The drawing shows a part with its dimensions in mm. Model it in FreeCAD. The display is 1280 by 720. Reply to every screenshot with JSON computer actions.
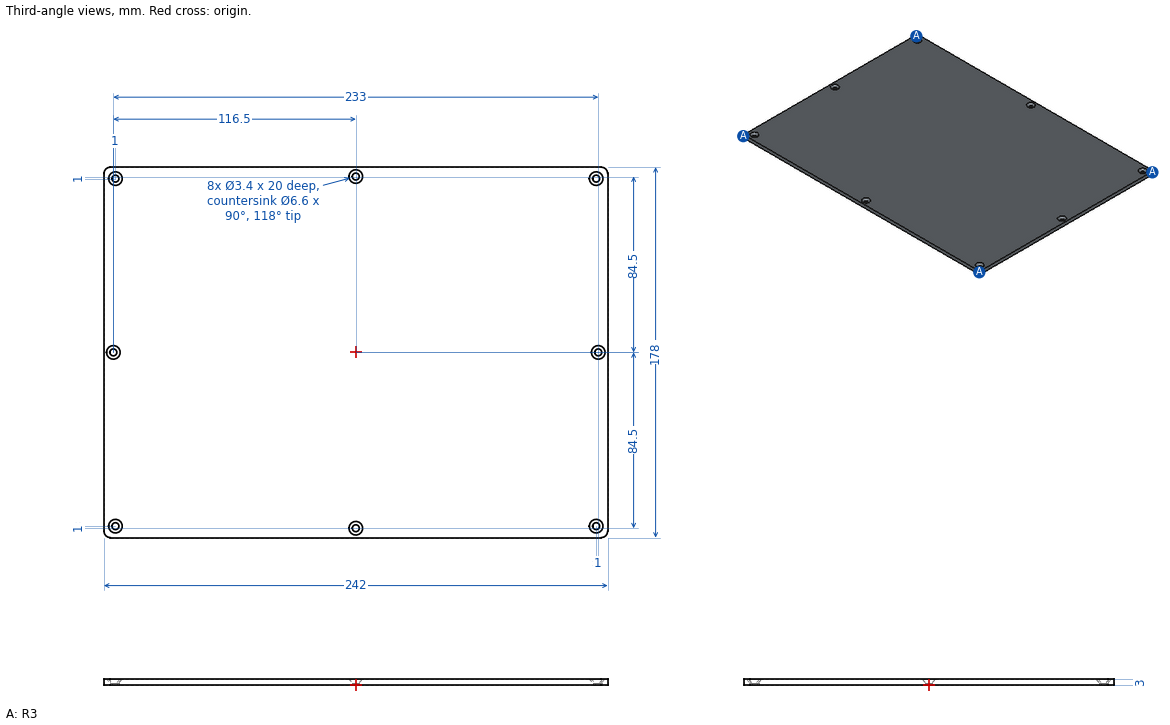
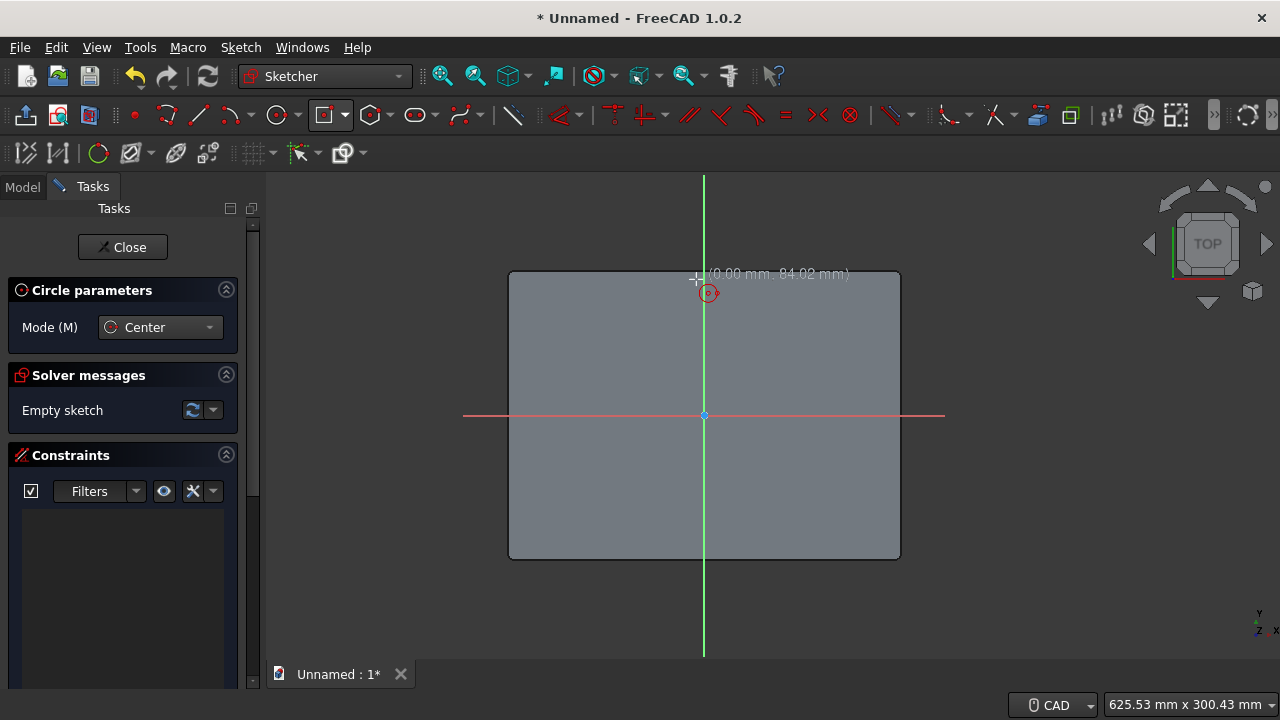
{"action": "left_click", "coordinate": [704, 279]}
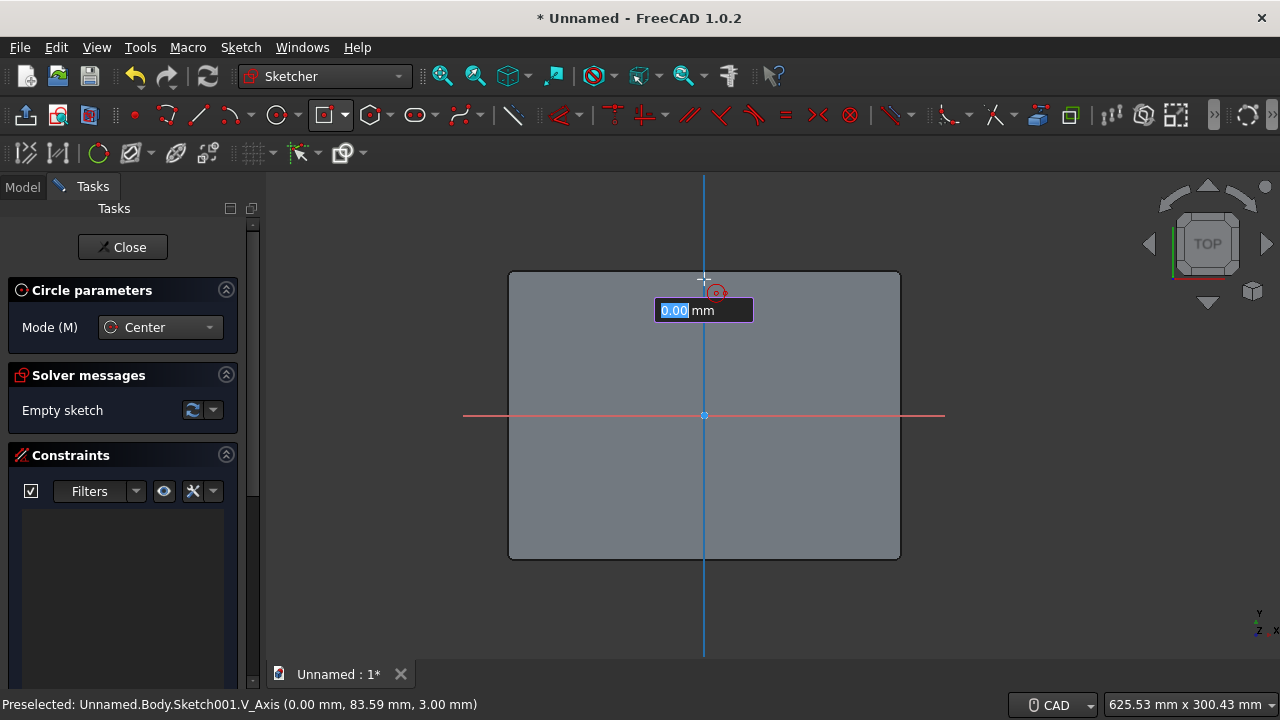
{"action": "scroll", "coordinate": [707, 278], "scroll_direction": "up", "scroll_amount": 10}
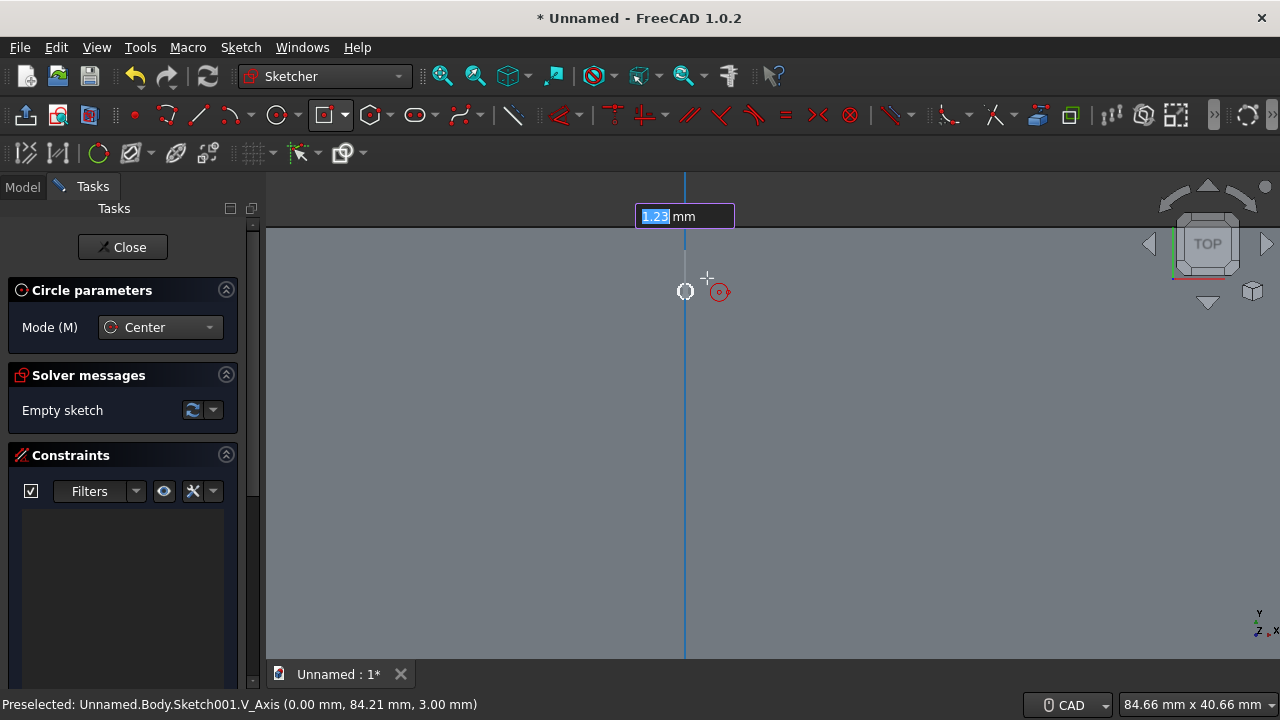
{"action": "left_click", "coordinate": [705, 274]}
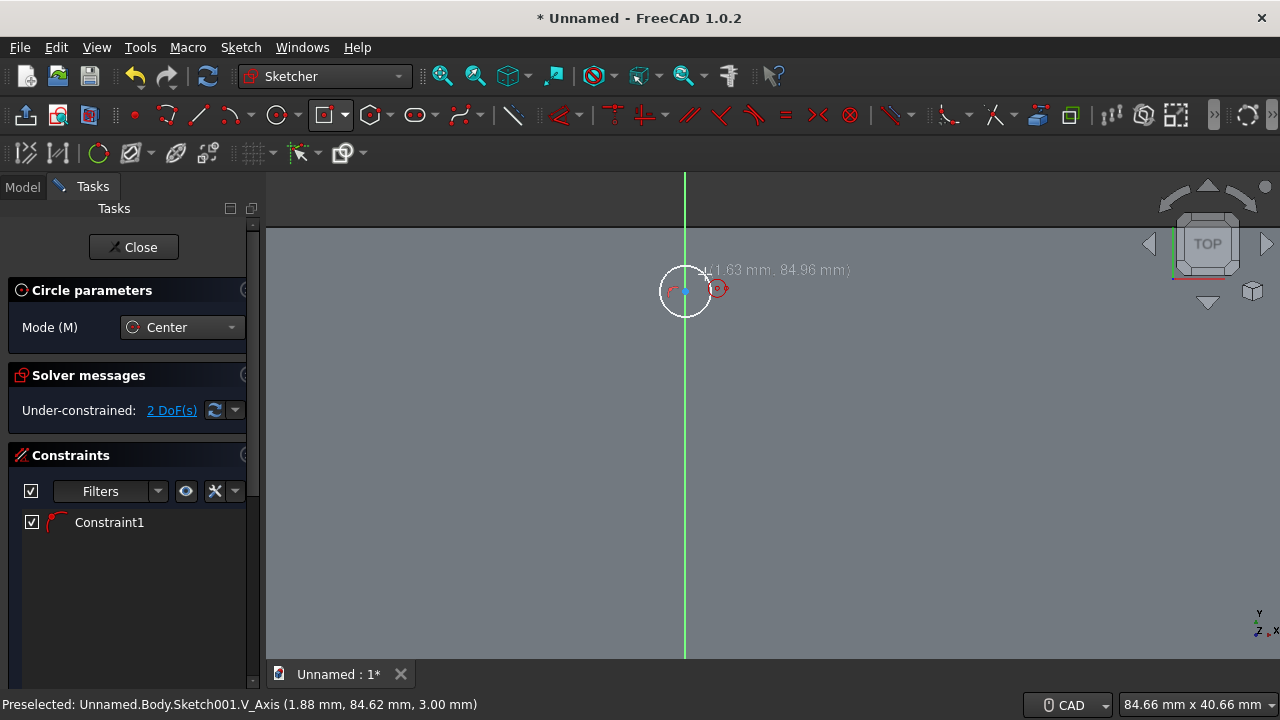
{"action": "scroll", "coordinate": [707, 278], "scroll_direction": "down", "scroll_amount": 10}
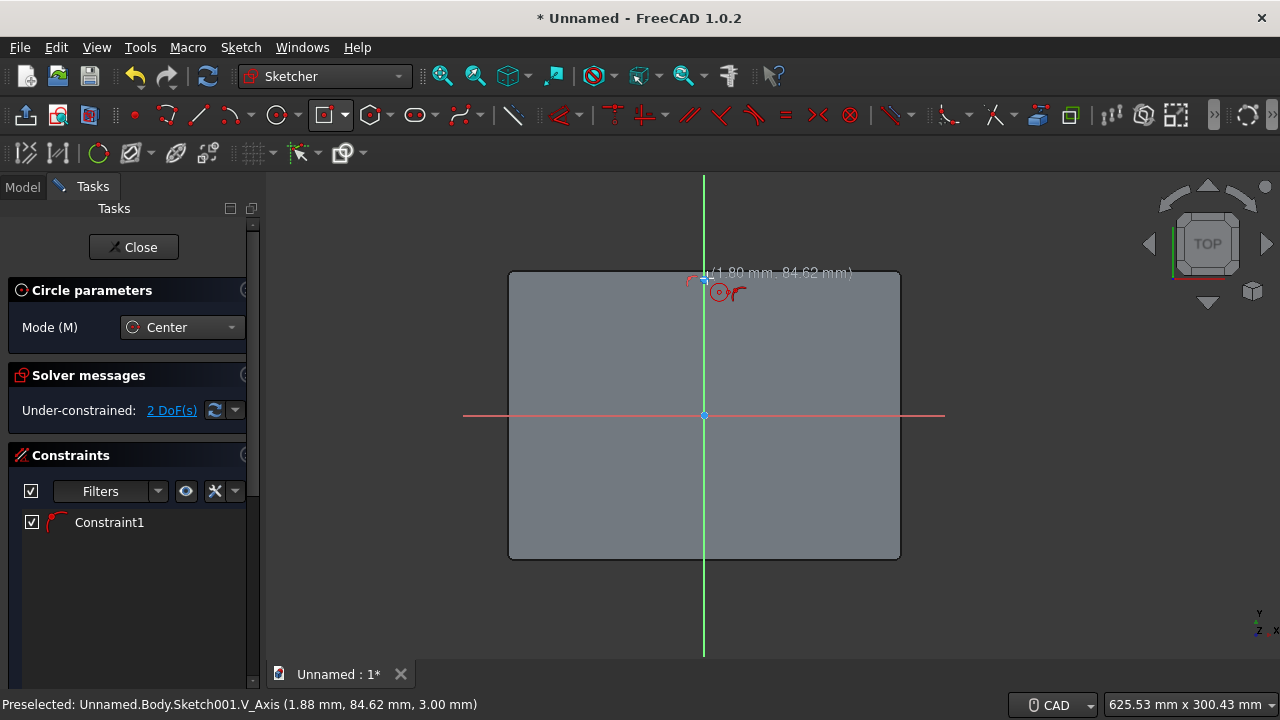
{"action": "scroll", "coordinate": [516, 415], "scroll_direction": "up", "scroll_amount": 11}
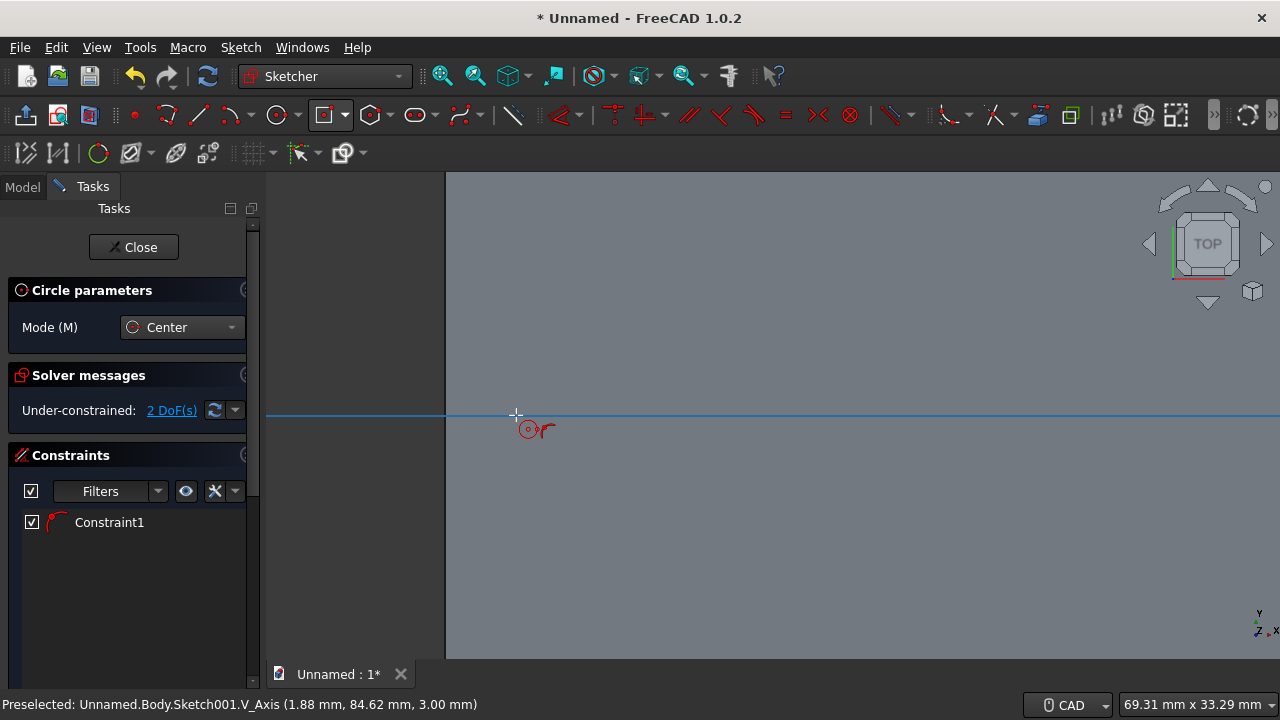
{"action": "scroll", "coordinate": [516, 416], "scroll_direction": "down", "scroll_amount": 11}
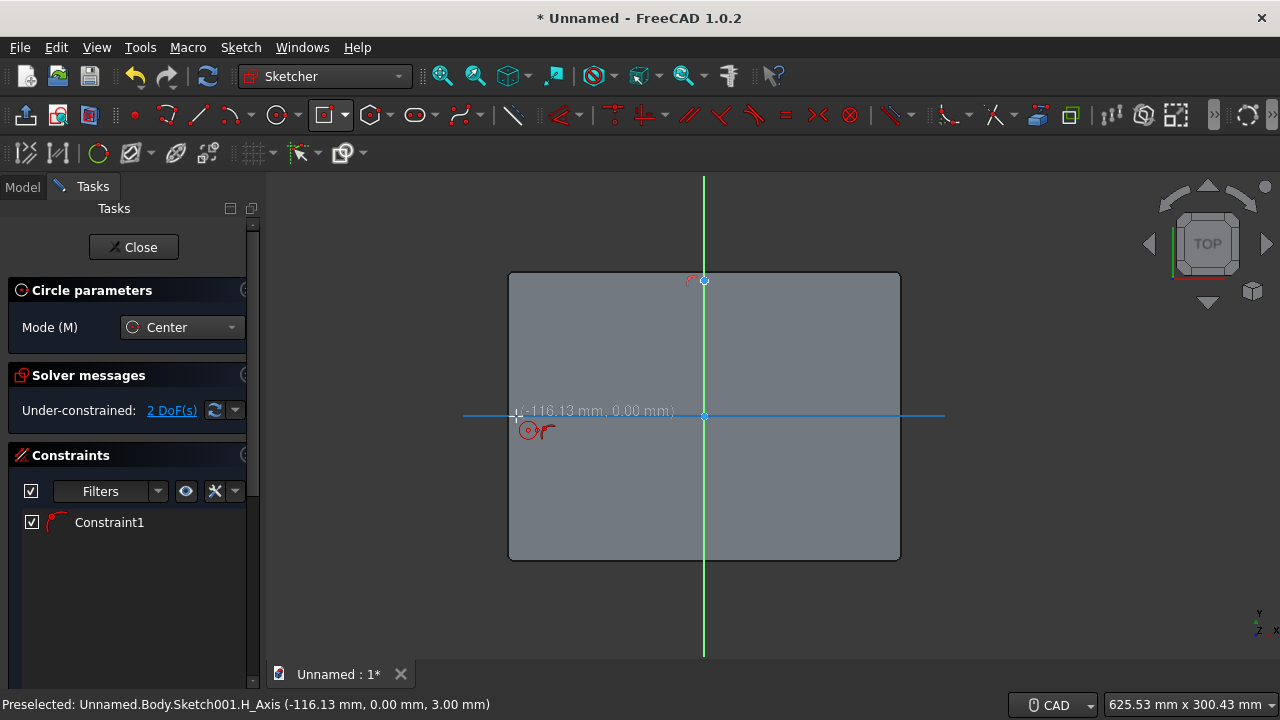
{"action": "left_click", "coordinate": [516, 416]}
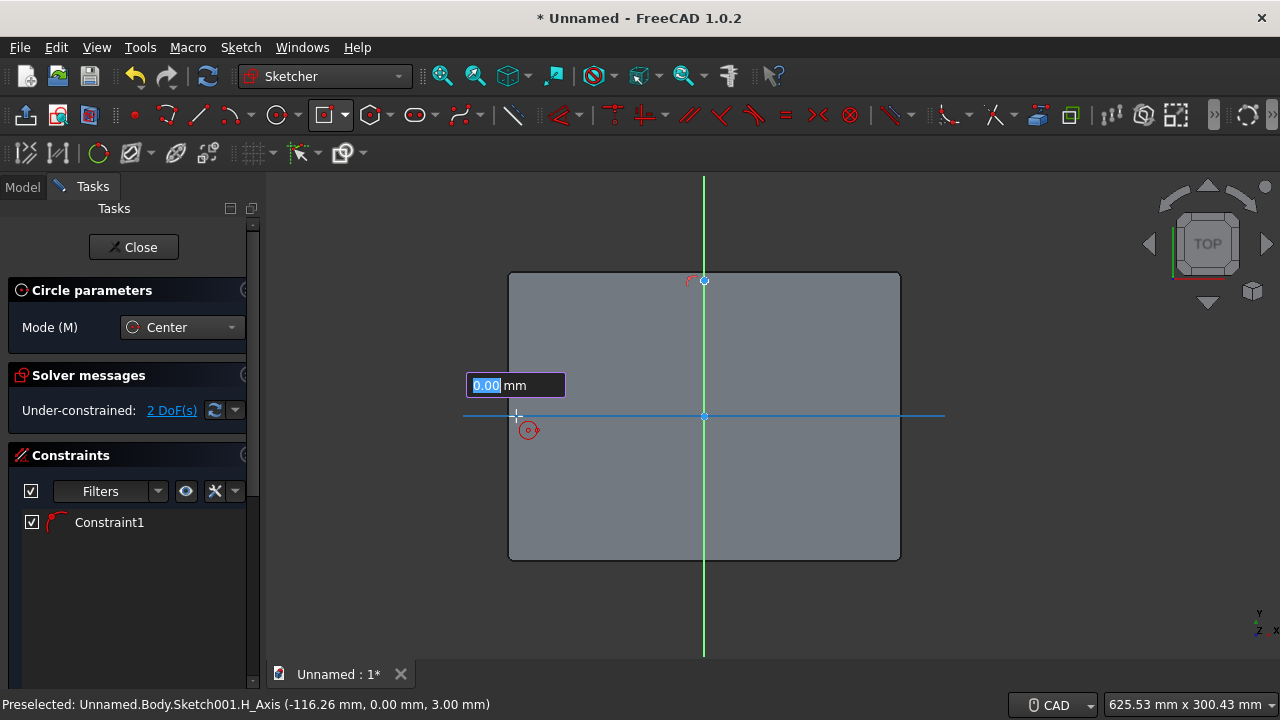
{"action": "scroll", "coordinate": [515, 419], "scroll_direction": "up", "scroll_amount": 10}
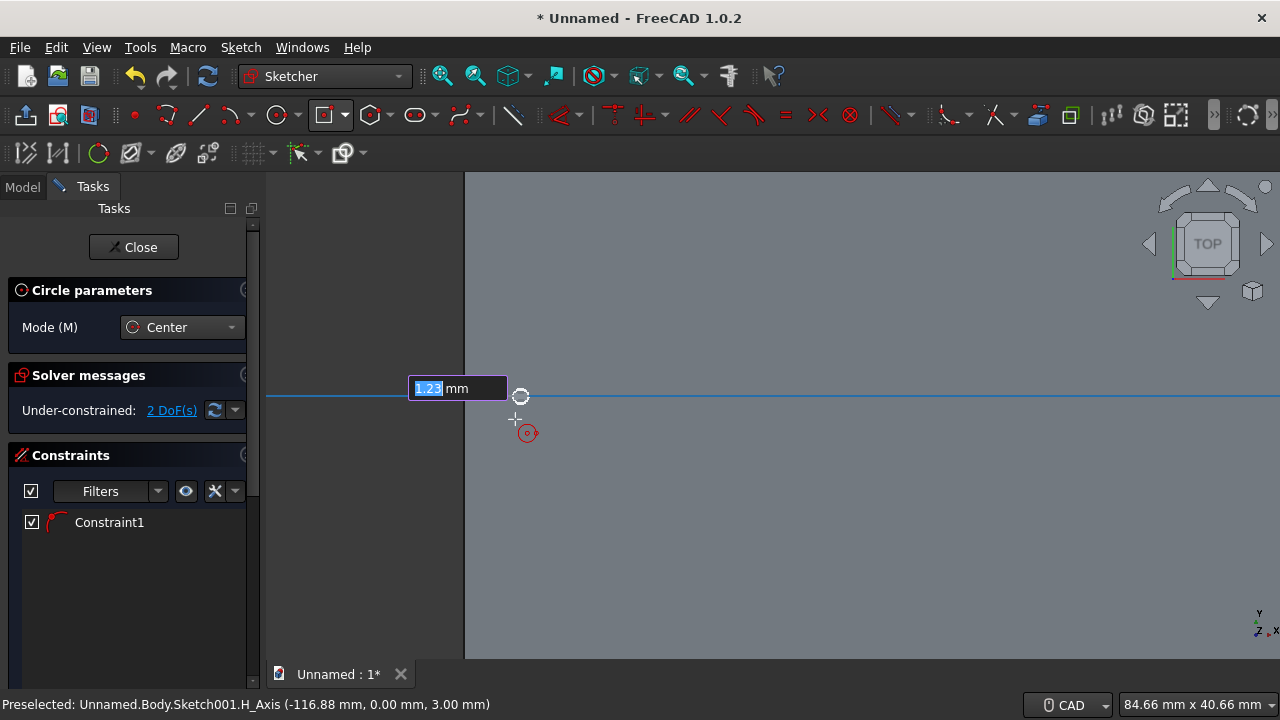
{"action": "left_click", "coordinate": [511, 416]}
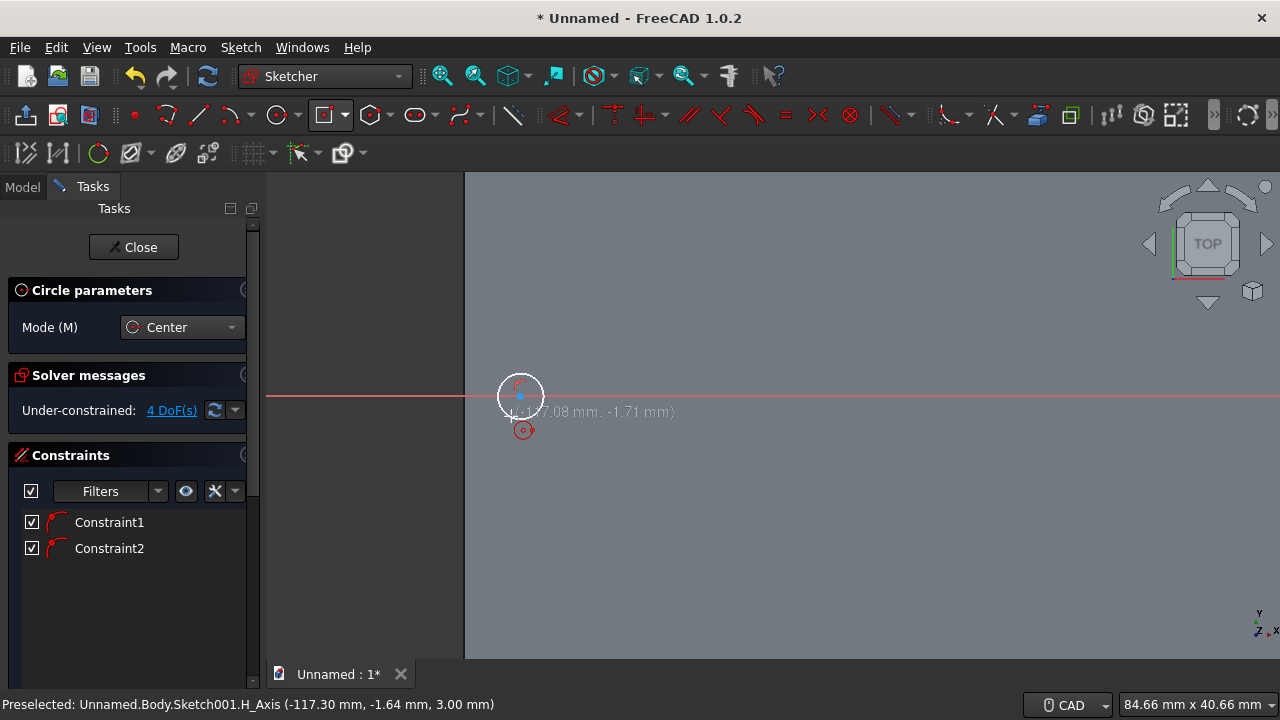
{"action": "scroll", "coordinate": [515, 418], "scroll_direction": "down", "scroll_amount": 10}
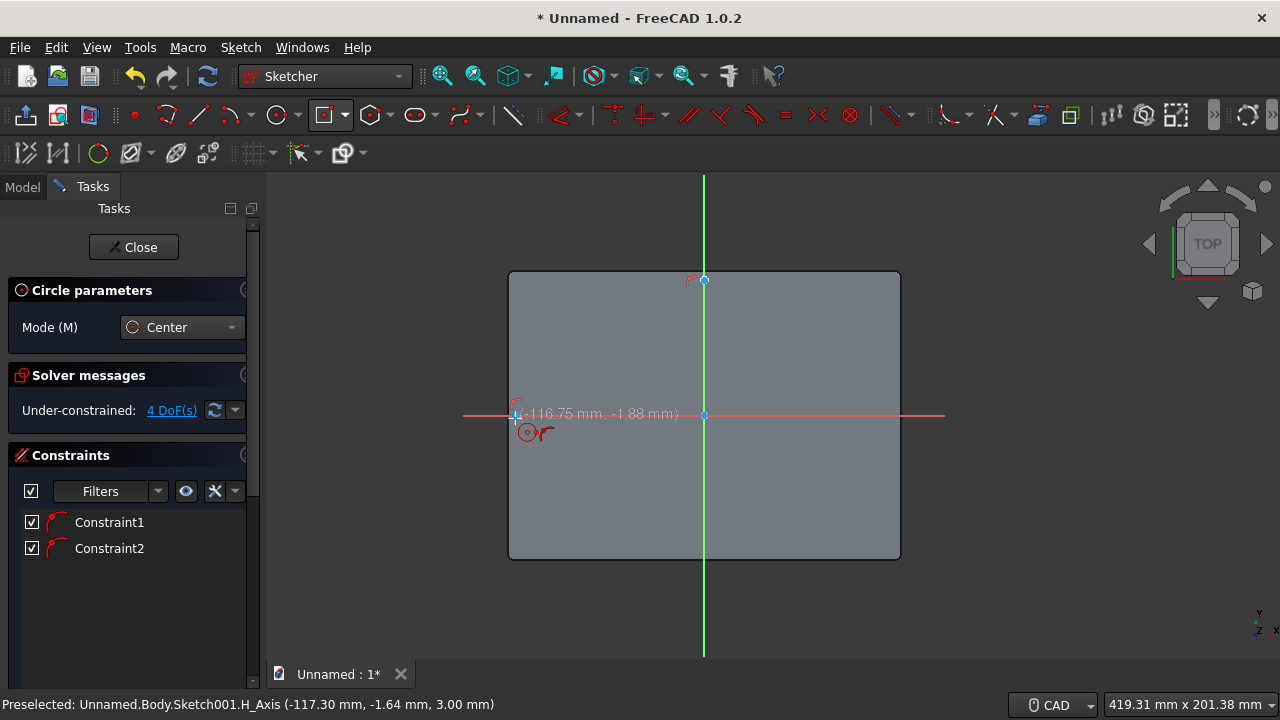
{"action": "scroll", "coordinate": [704, 553], "scroll_direction": "up", "scroll_amount": 11}